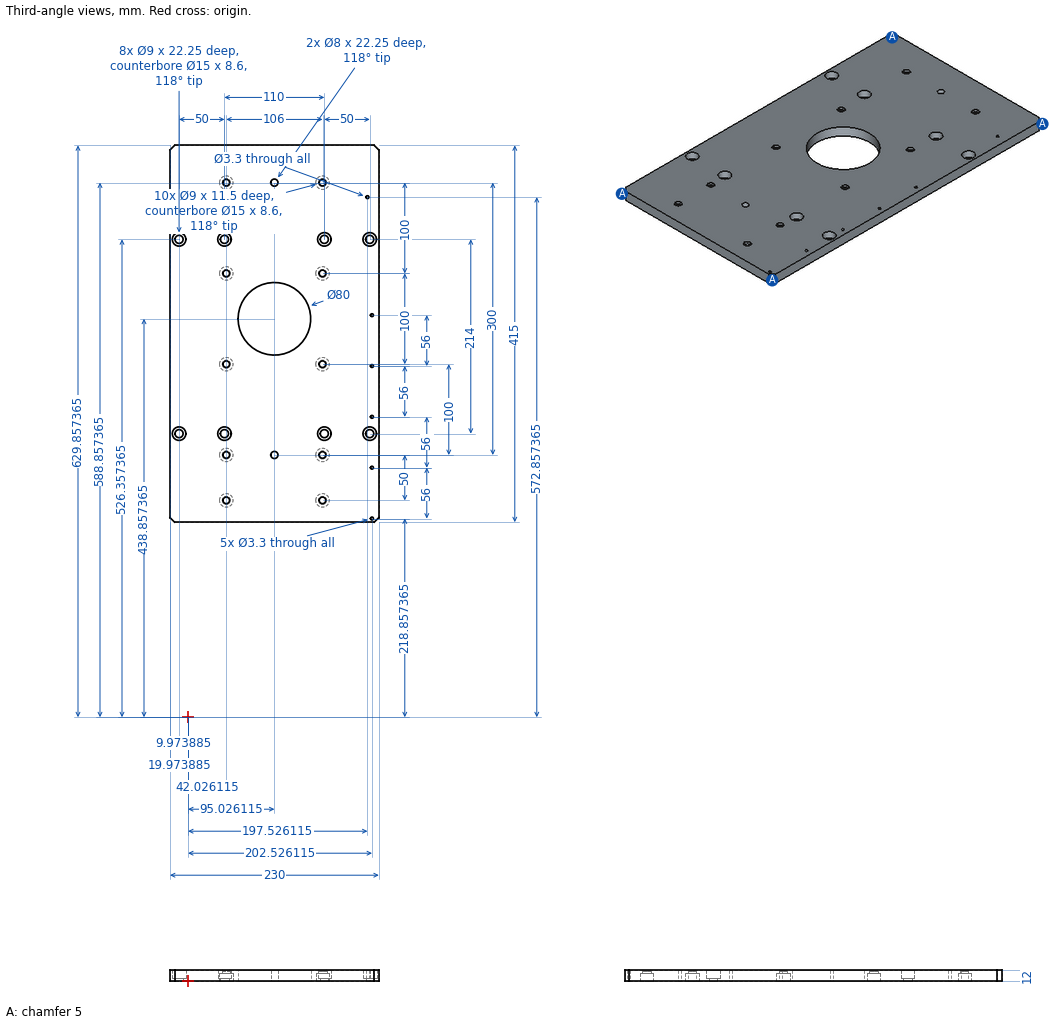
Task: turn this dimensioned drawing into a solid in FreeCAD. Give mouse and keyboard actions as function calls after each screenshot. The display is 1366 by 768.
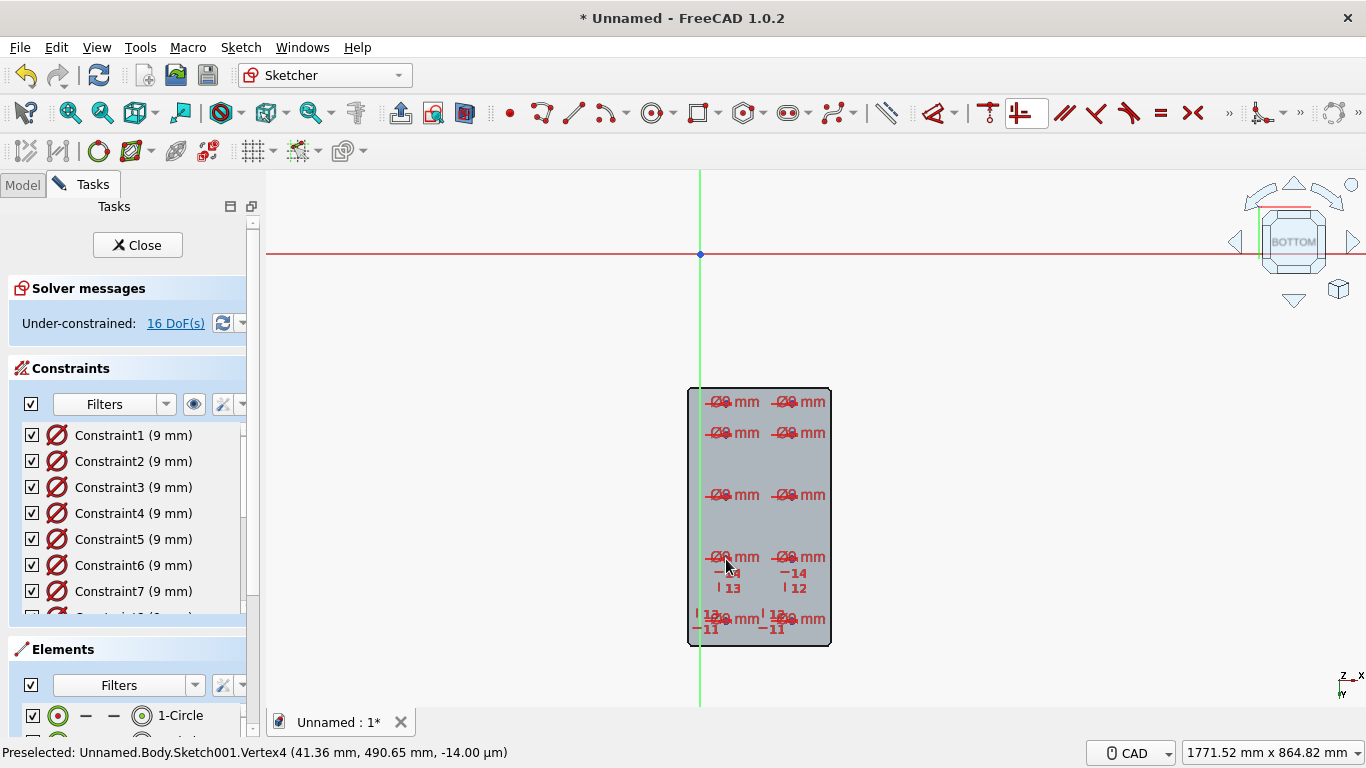
click(792, 559)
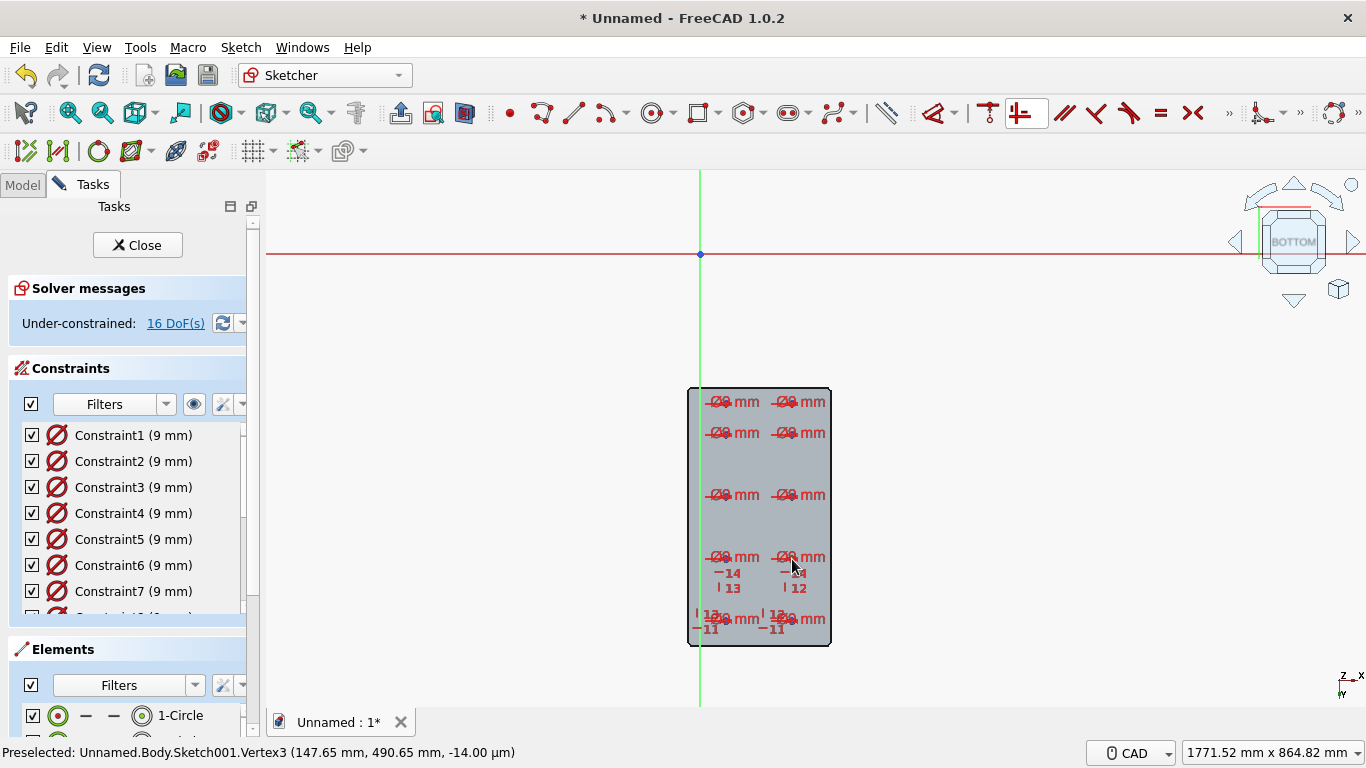
click(792, 497)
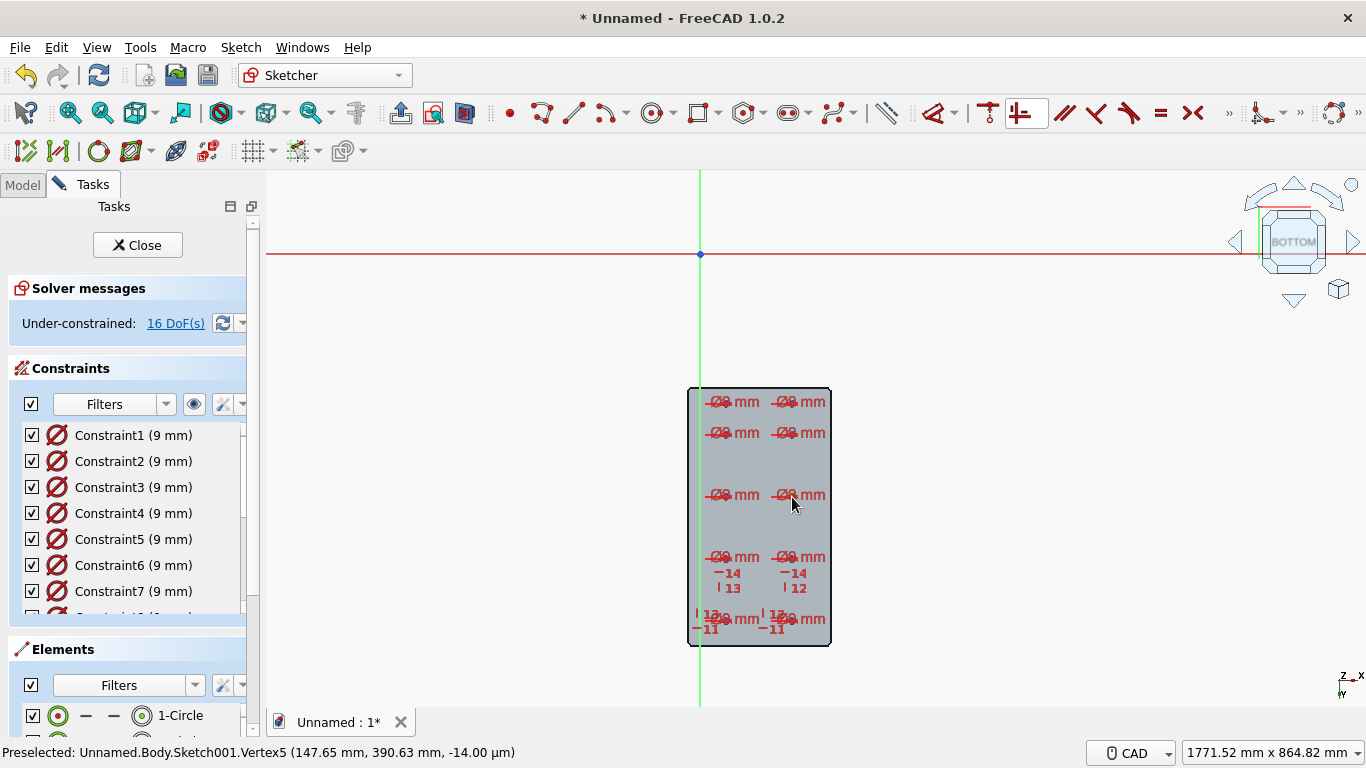
click(1042, 114)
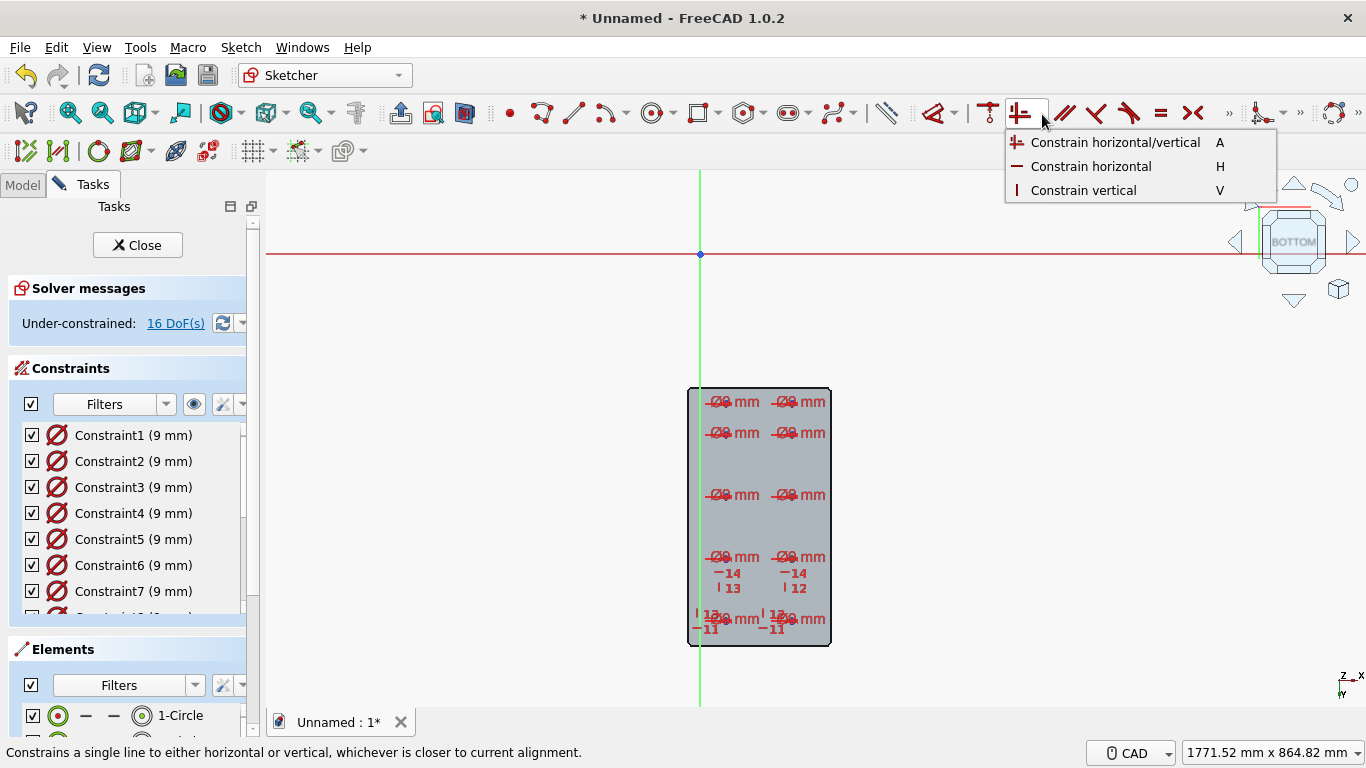
click(1141, 190)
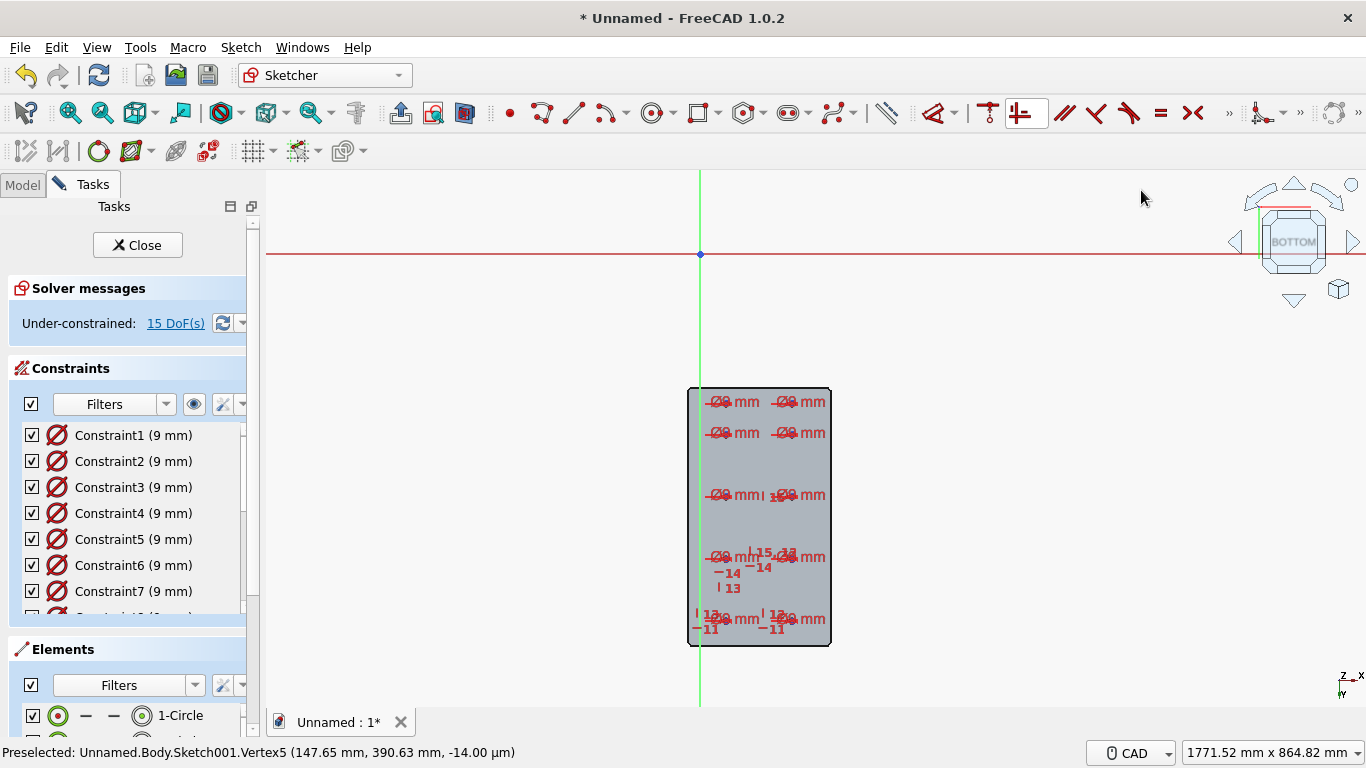
click(726, 559)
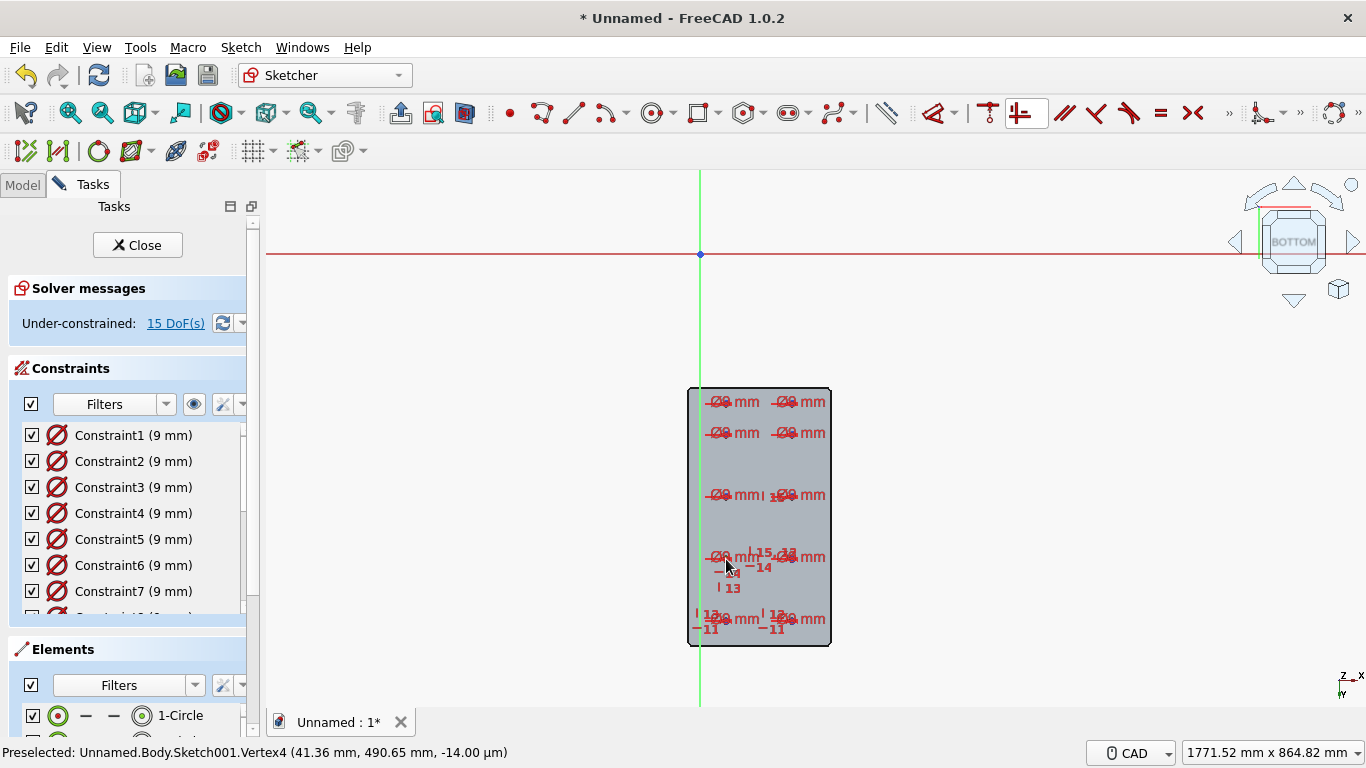
click(726, 497)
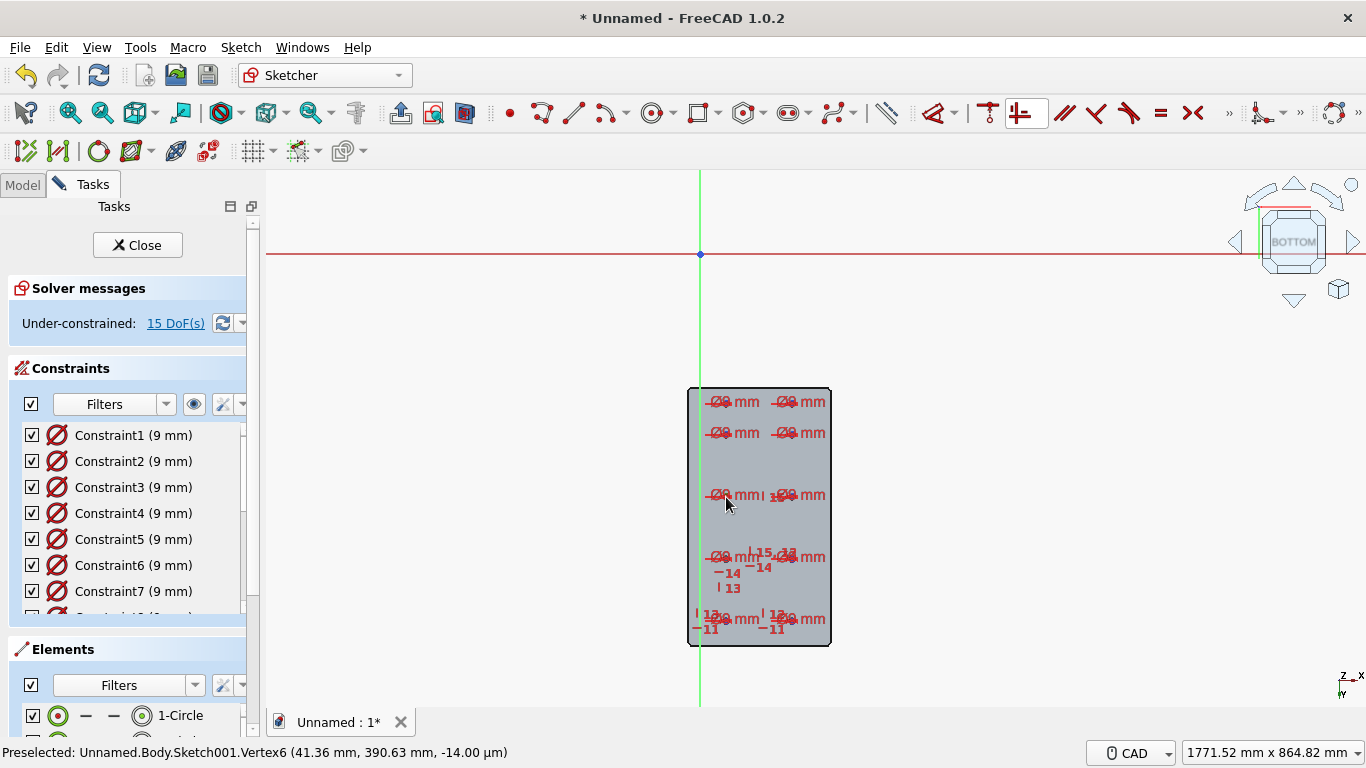
click(1042, 114)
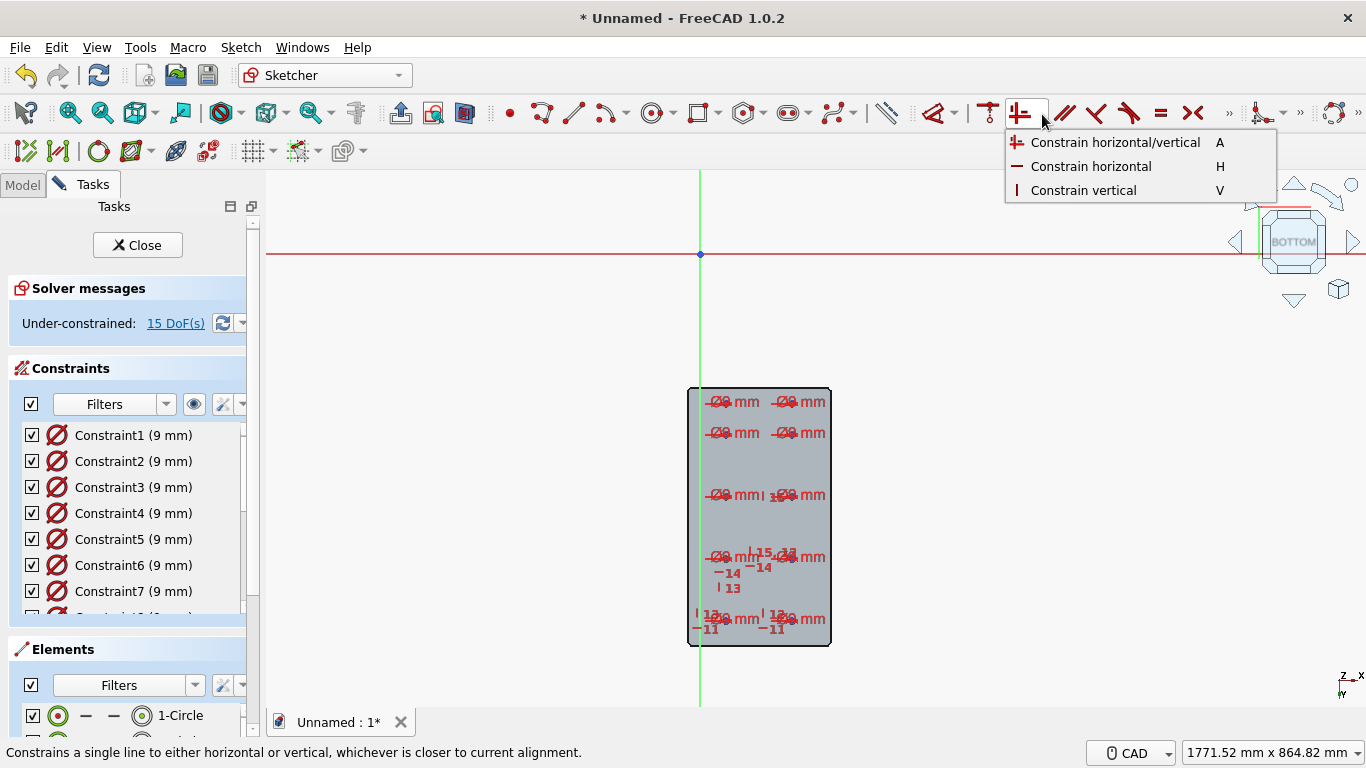
click(1141, 190)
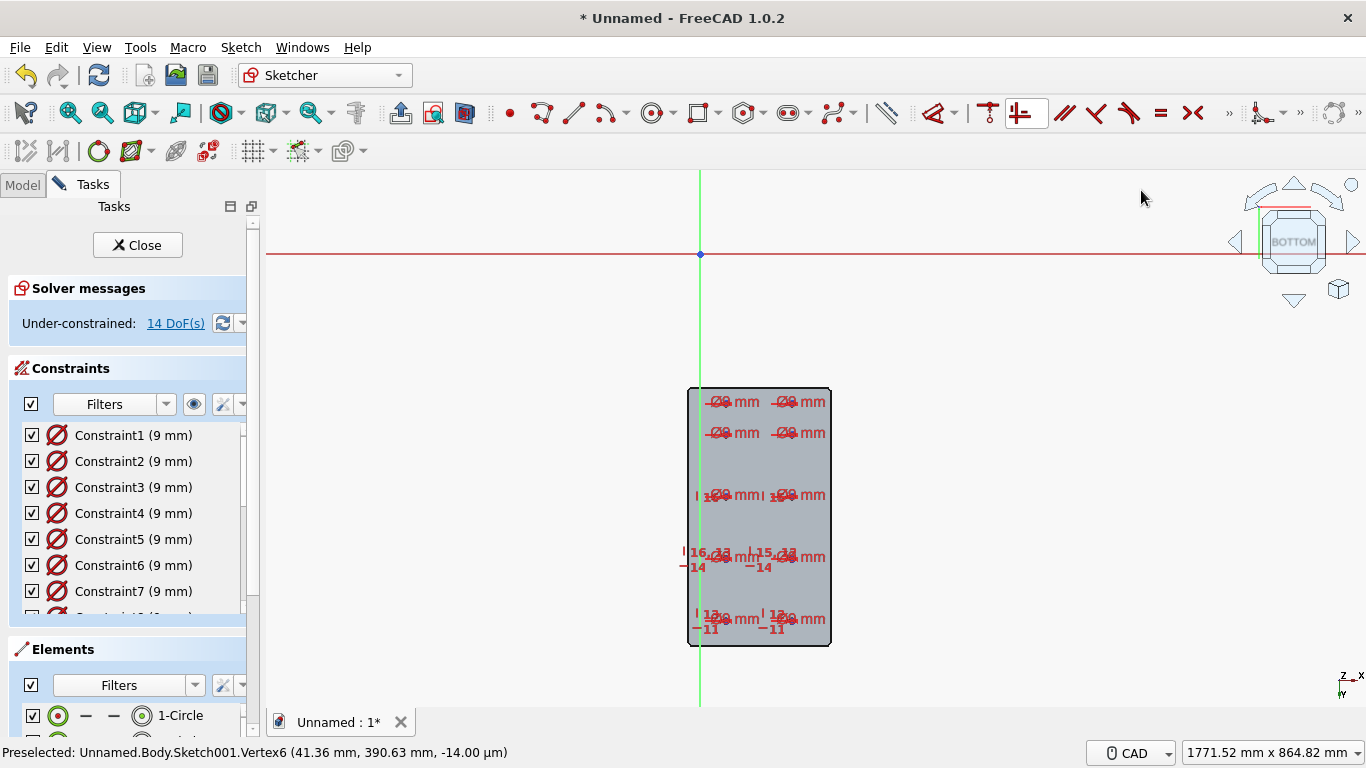
click(792, 497)